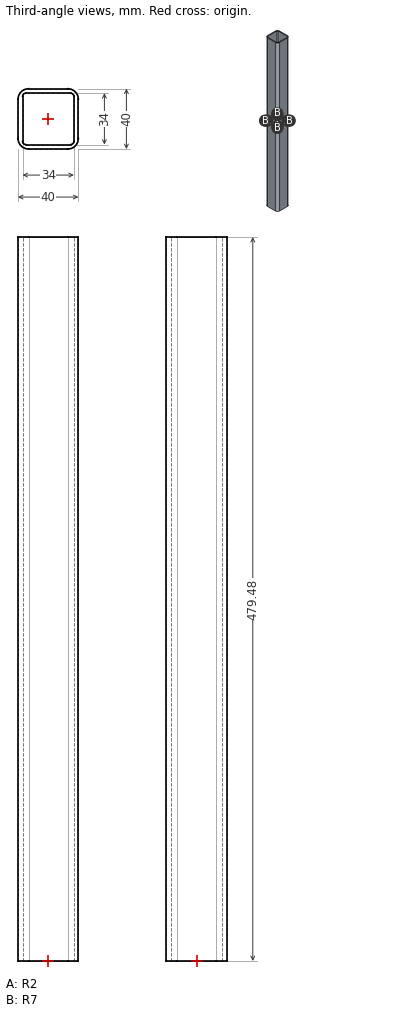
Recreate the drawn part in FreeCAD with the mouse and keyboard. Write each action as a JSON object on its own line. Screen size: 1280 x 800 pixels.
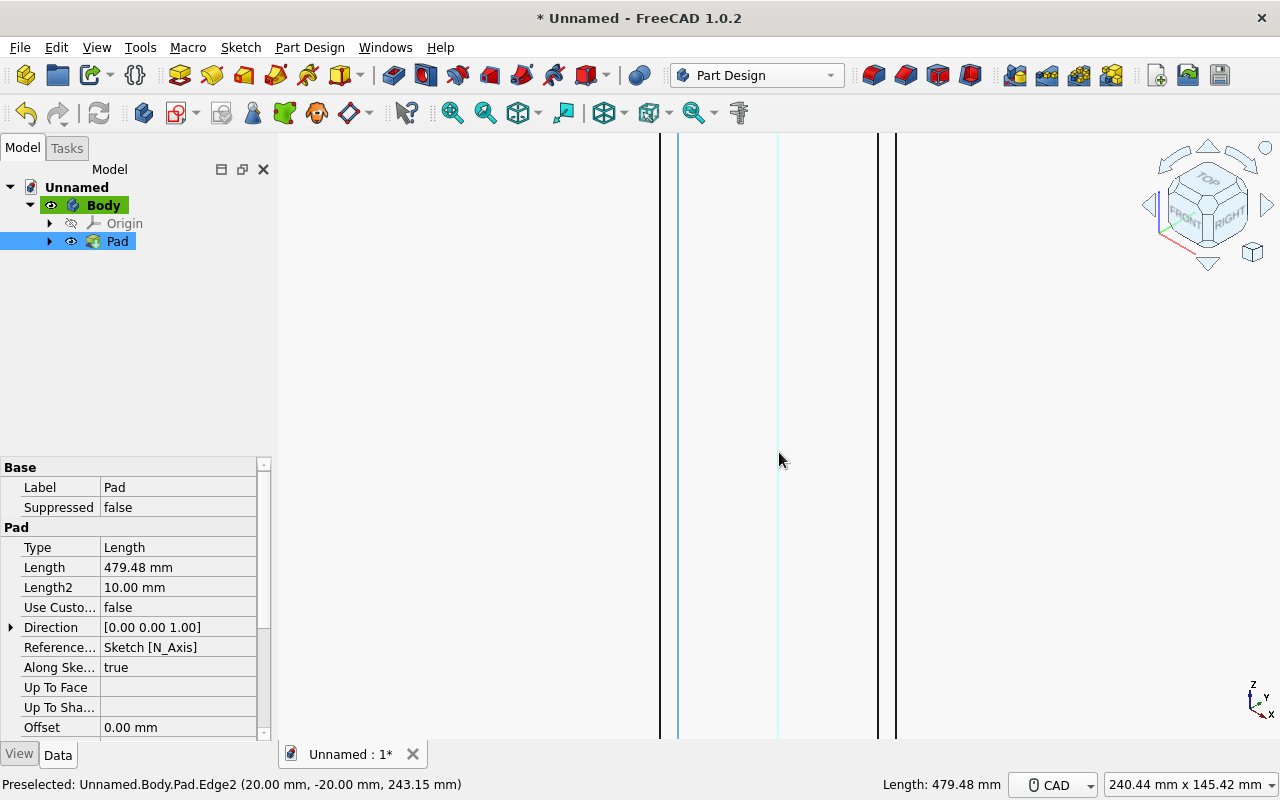
{"action": "left_click", "coordinate": [878, 397], "text": "ctrl"}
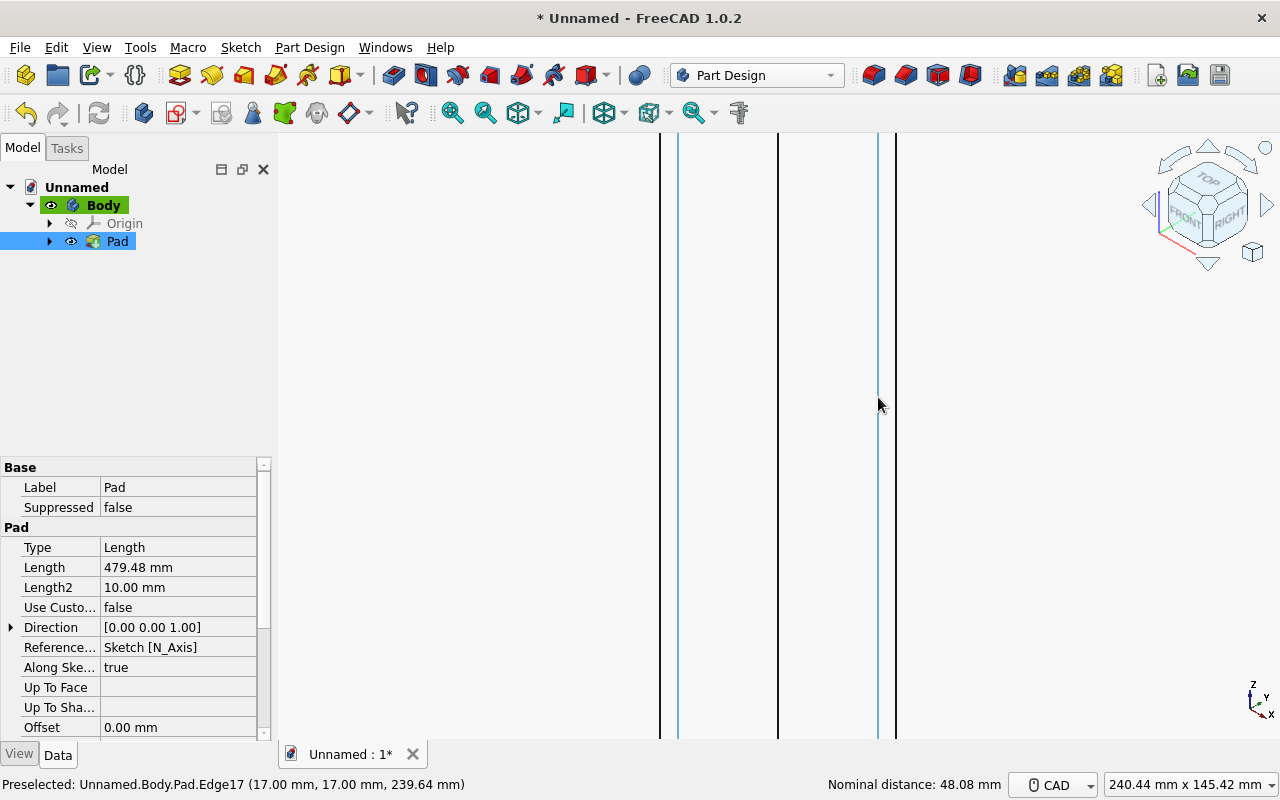
{"action": "key", "text": "v f"}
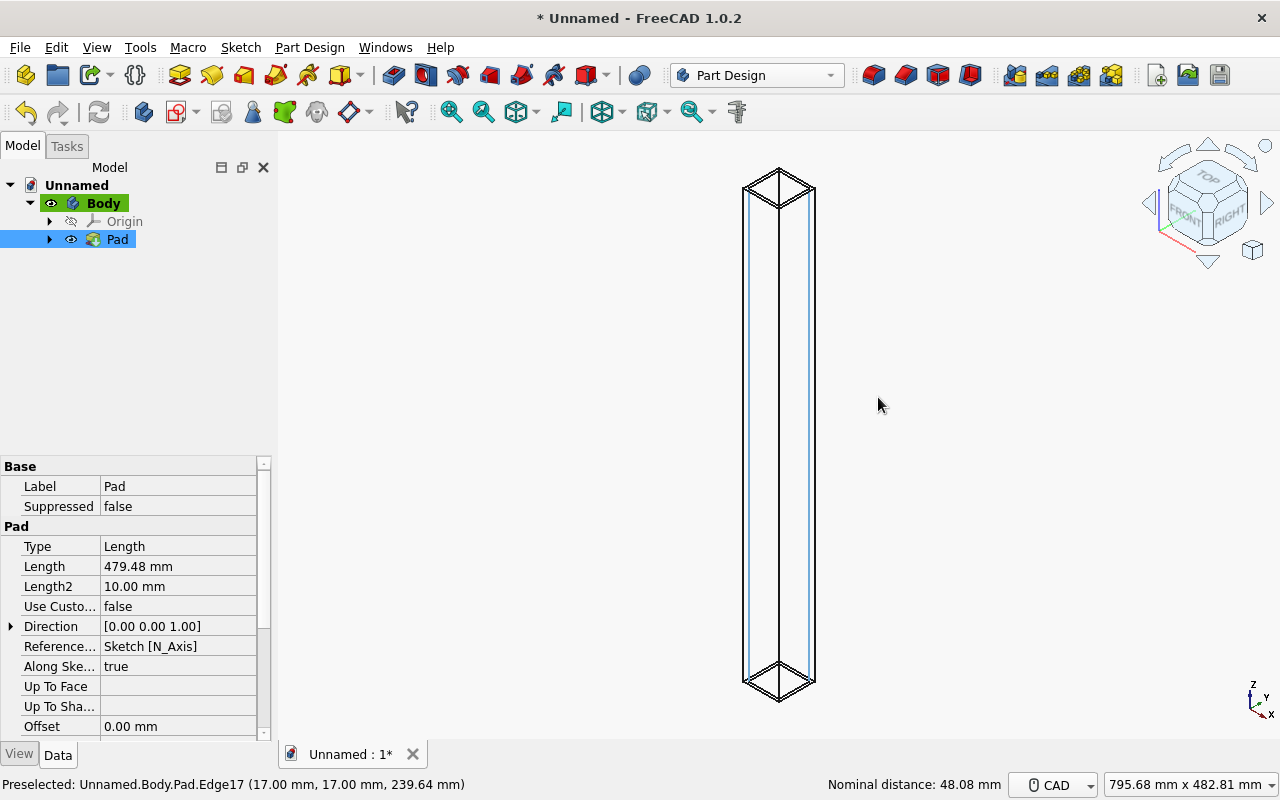
{"action": "key", "text": "2"}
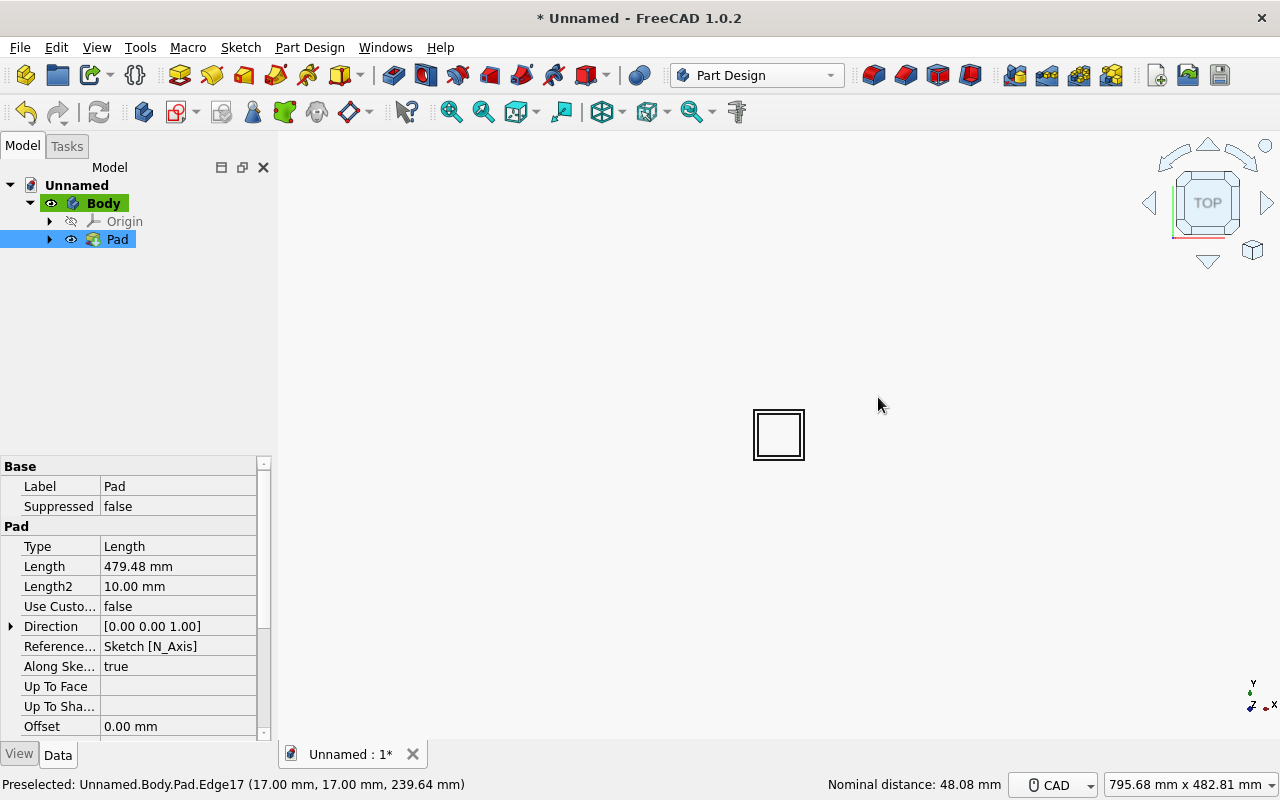
{"action": "left_click", "coordinate": [452, 112]}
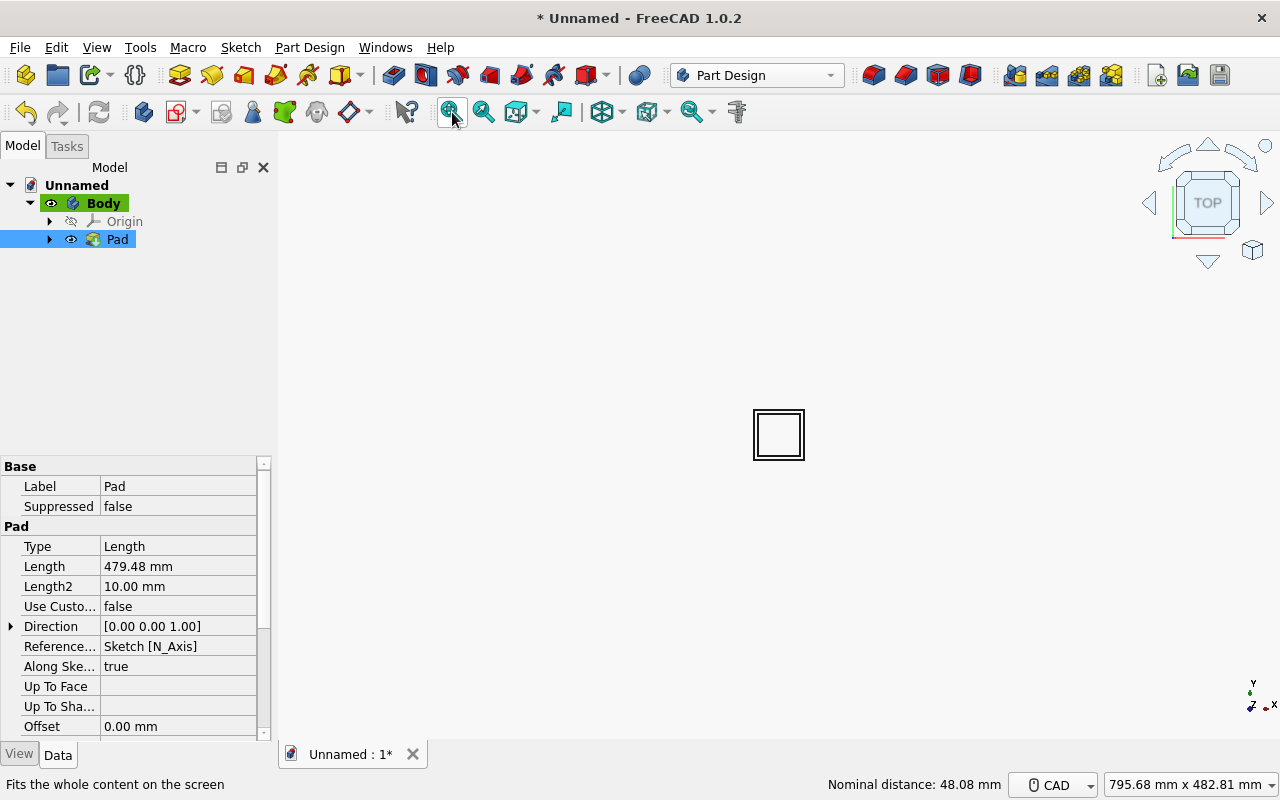
{"action": "scroll", "coordinate": [800, 455], "scroll_direction": "up", "scroll_amount": 6}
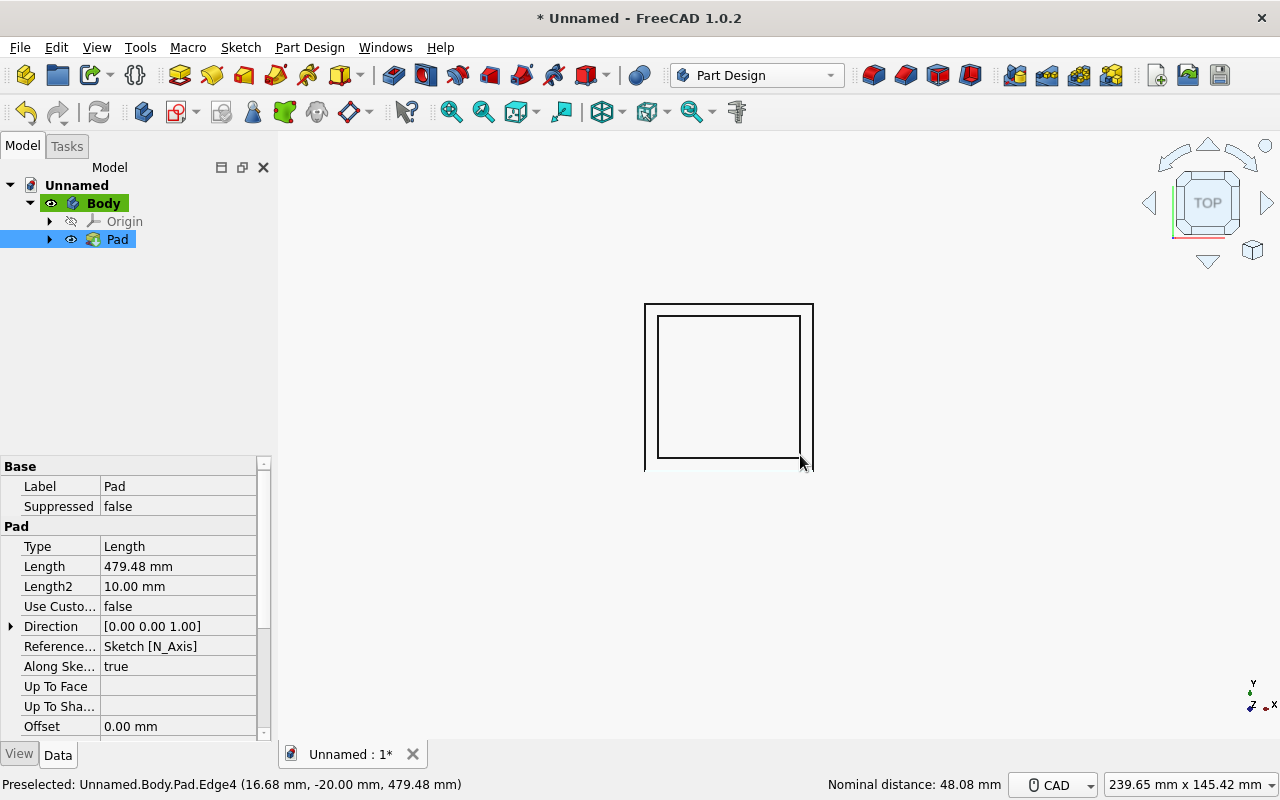
{"action": "key", "text": "v f"}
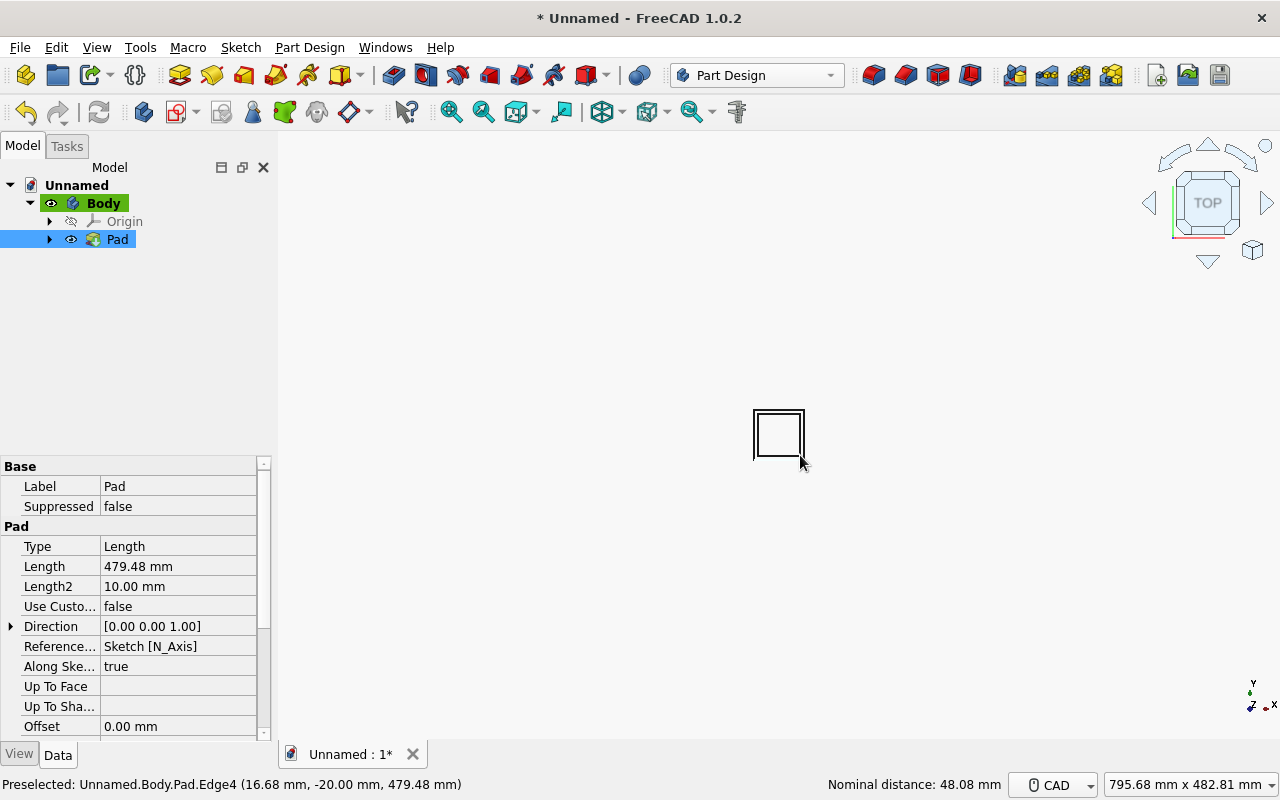
{"action": "key", "text": "1"}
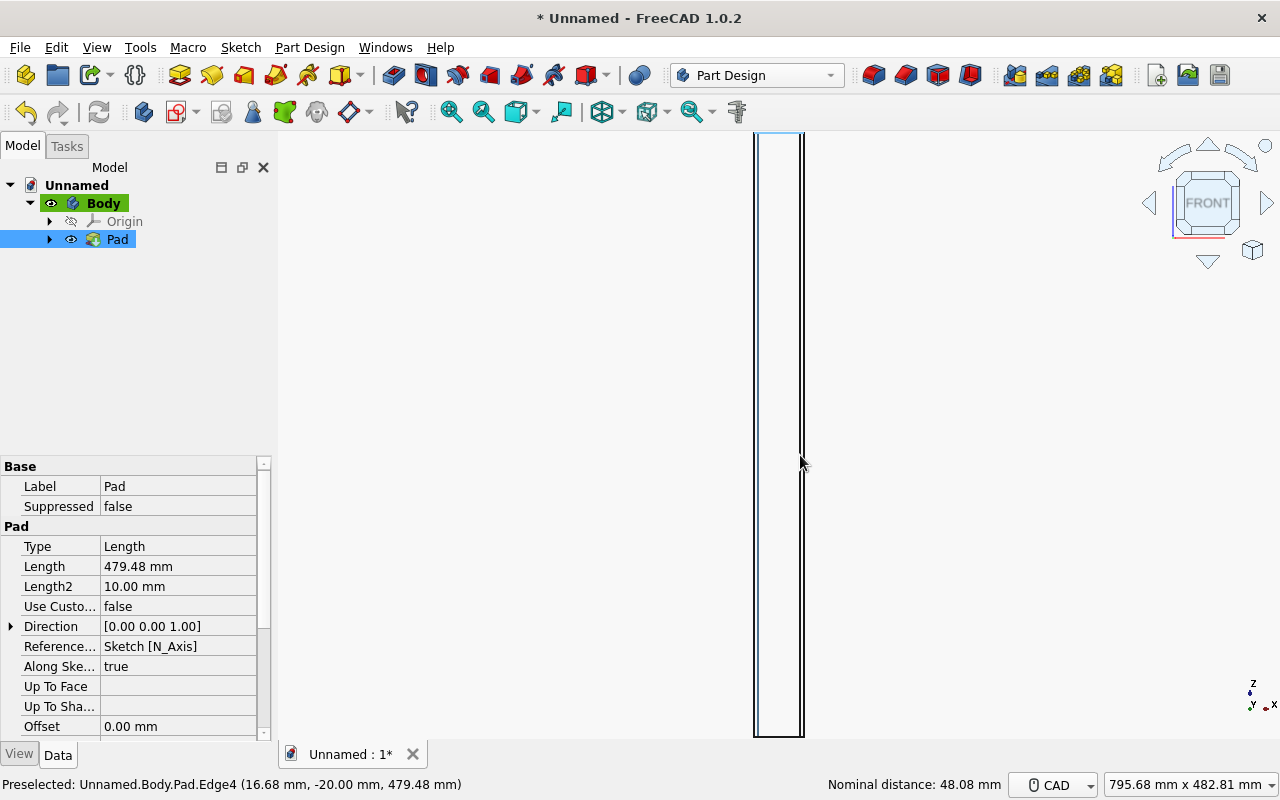
{"action": "scroll", "coordinate": [800, 434], "scroll_direction": "up", "scroll_amount": 6}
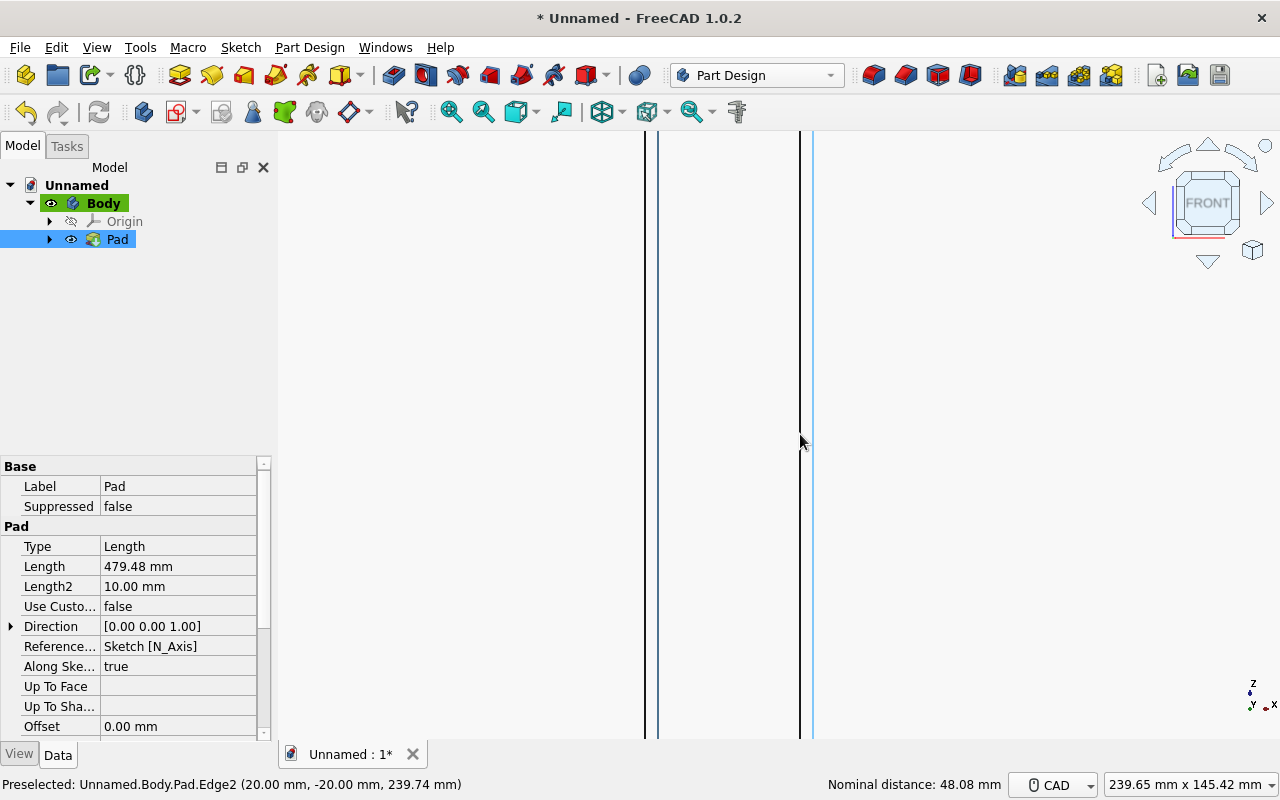
{"action": "left_click", "coordinate": [800, 435], "text": "ctrl"}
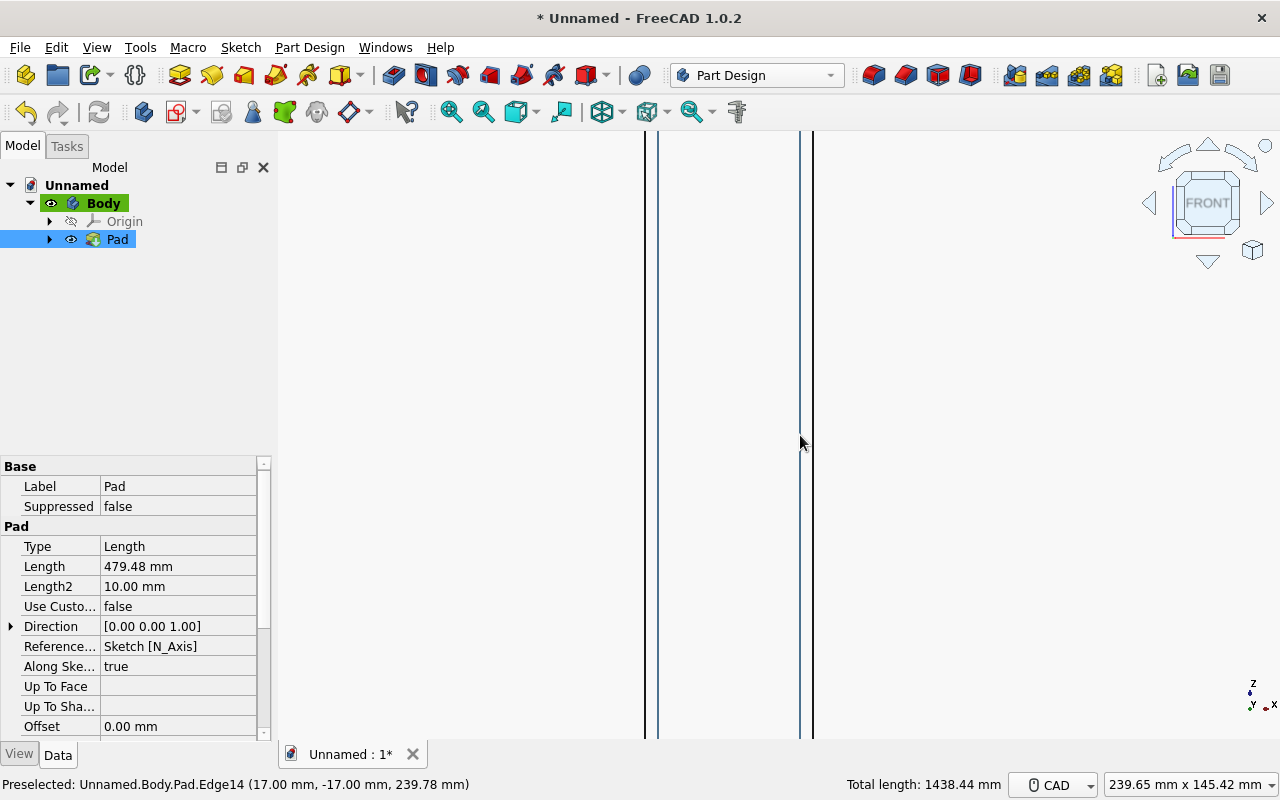
{"action": "left_click", "coordinate": [452, 112]}